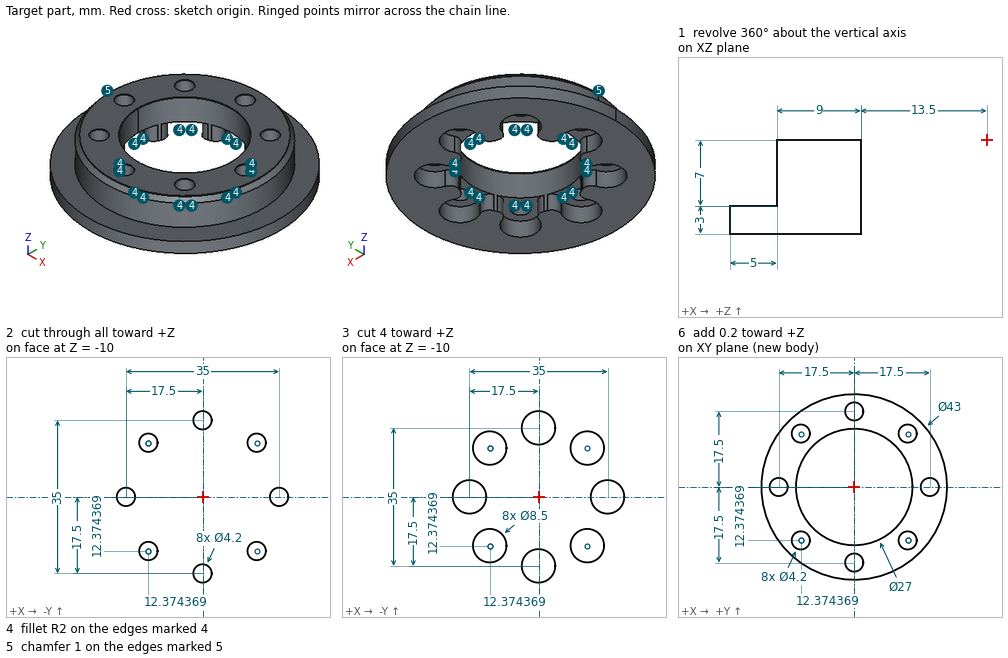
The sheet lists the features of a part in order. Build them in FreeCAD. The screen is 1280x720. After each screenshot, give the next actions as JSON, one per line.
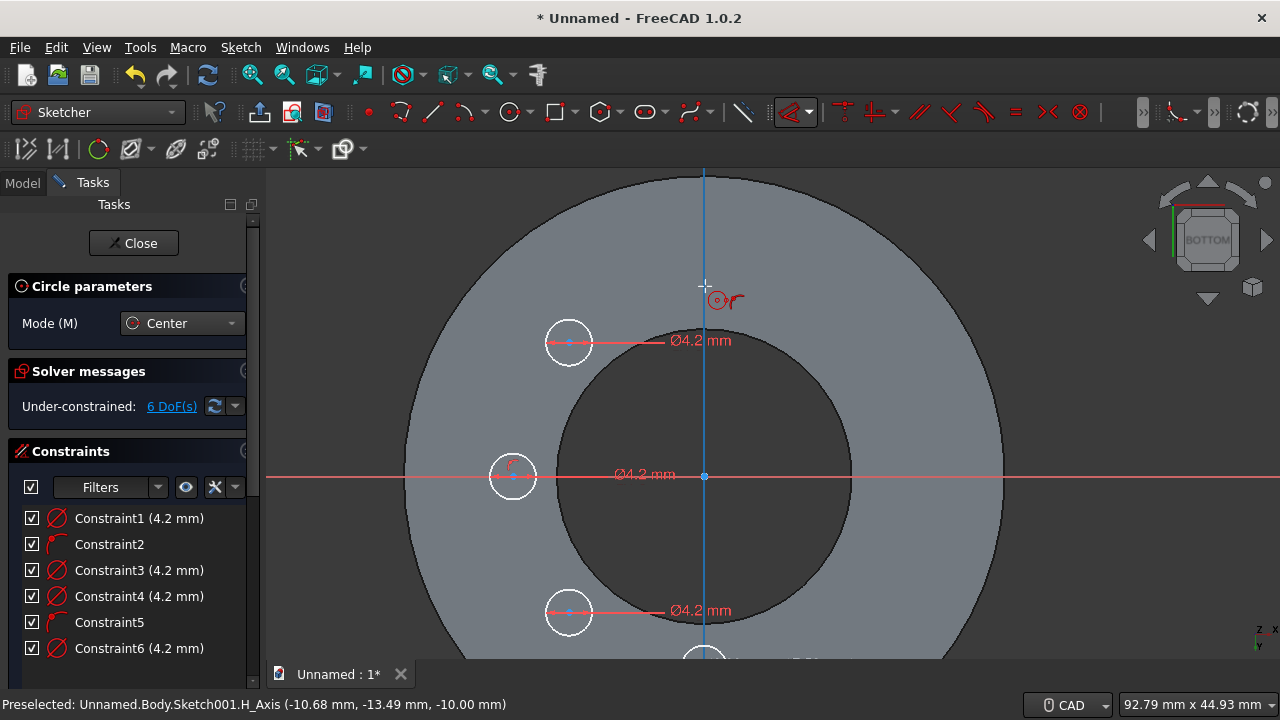
{"action": "left_click", "coordinate": [704, 285]}
{"action": "mouse_move", "coordinate": [720, 269]}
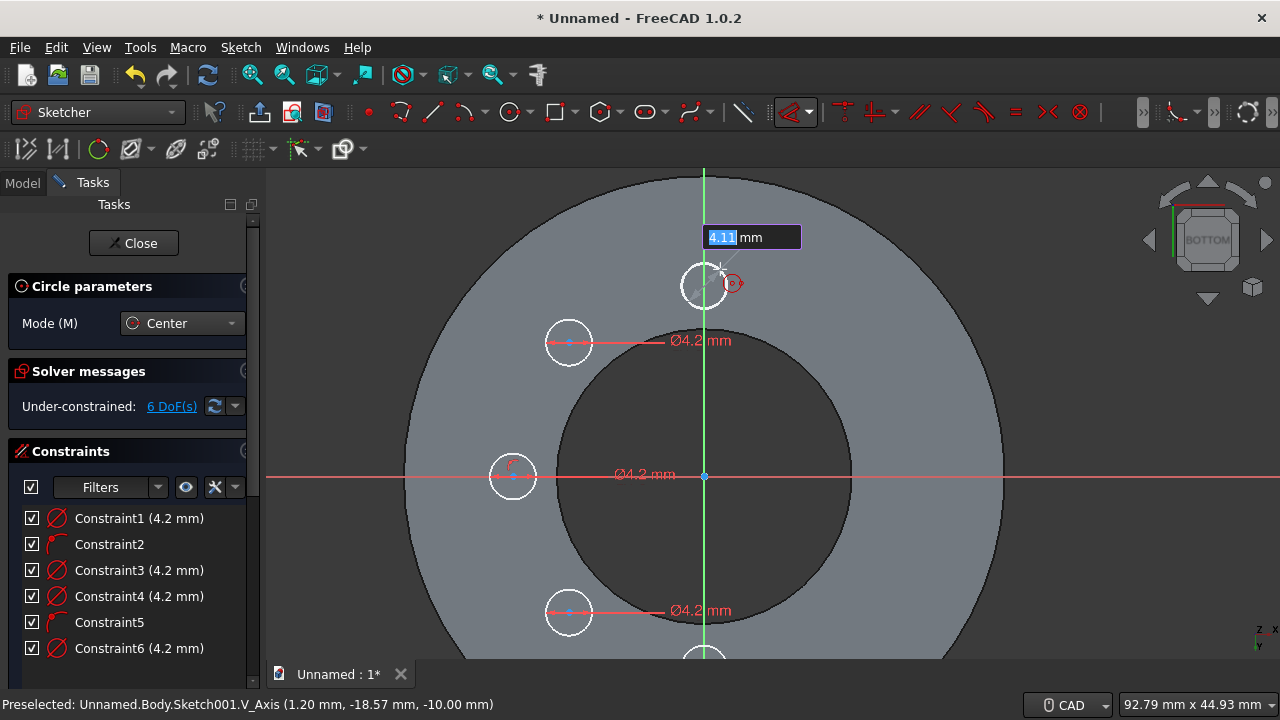
{"action": "type", "text": "4.2"}
{"action": "key", "text": "Return"}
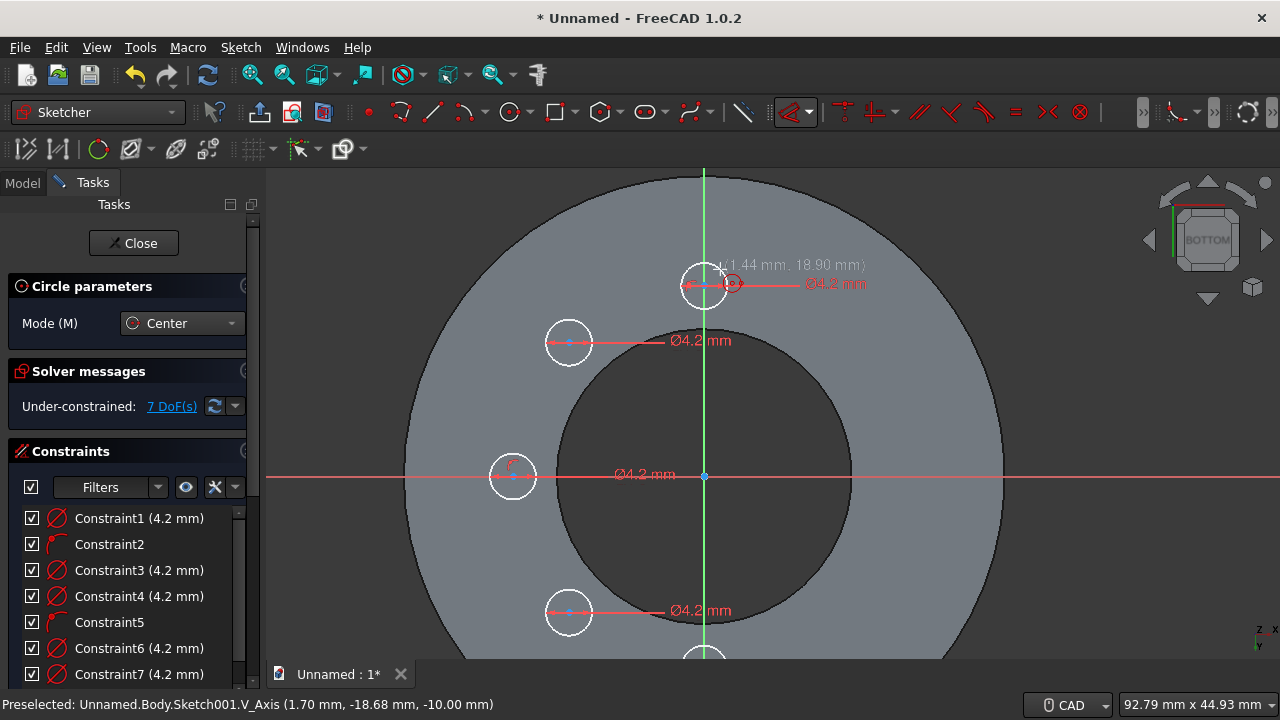
{"action": "left_click", "coordinate": [839, 341]}
{"action": "mouse_move", "coordinate": [856, 325]}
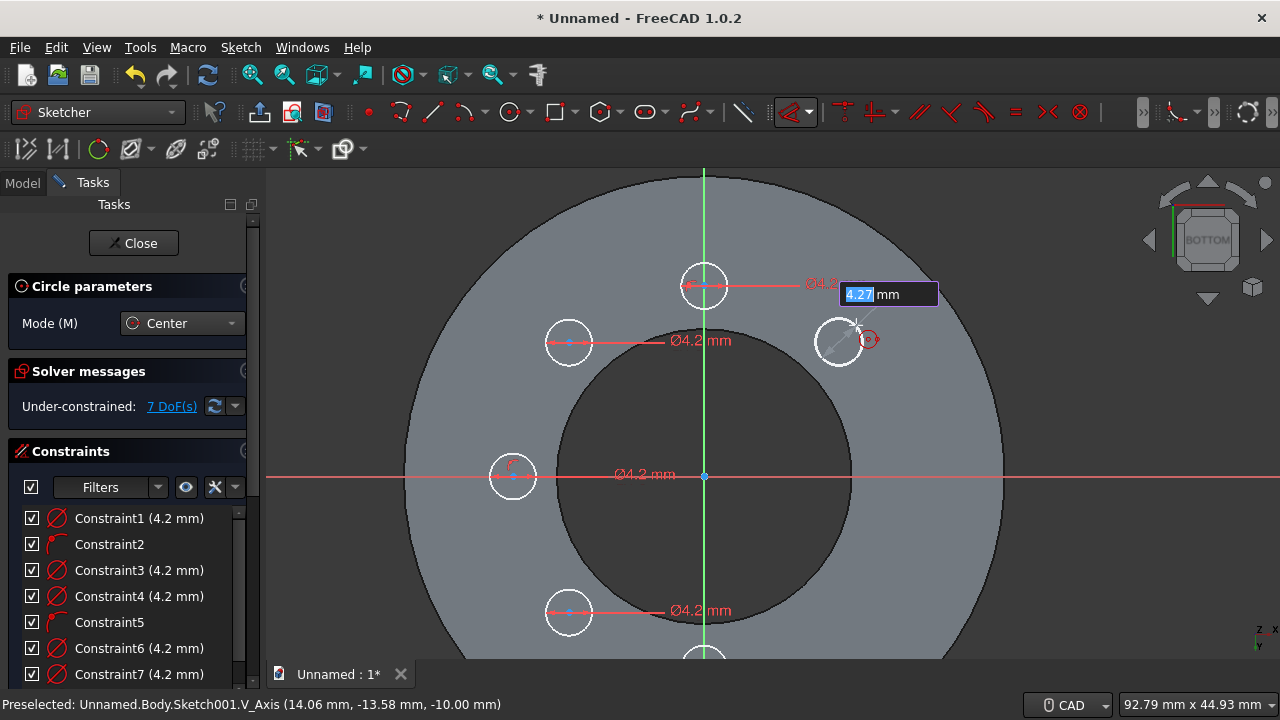
{"action": "type", "text": "4.2"}
{"action": "key", "text": "Return"}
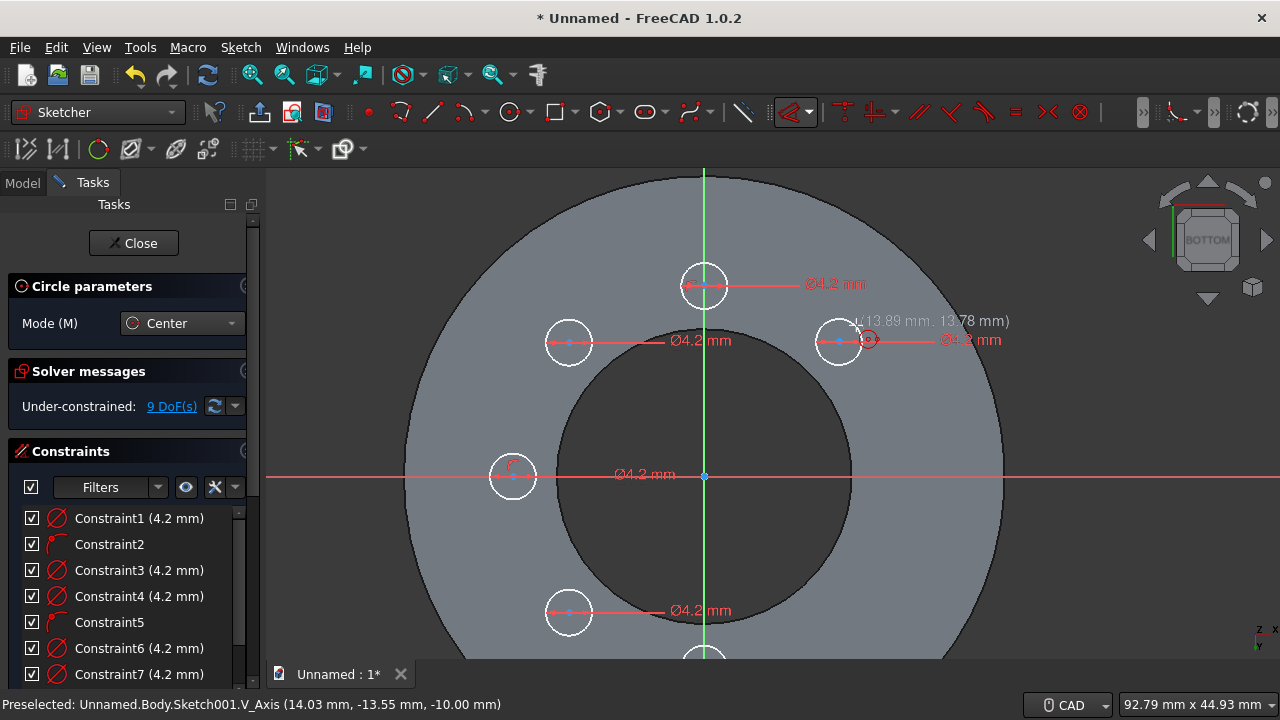
{"action": "left_click", "coordinate": [895, 477]}
{"action": "mouse_move", "coordinate": [912, 460]}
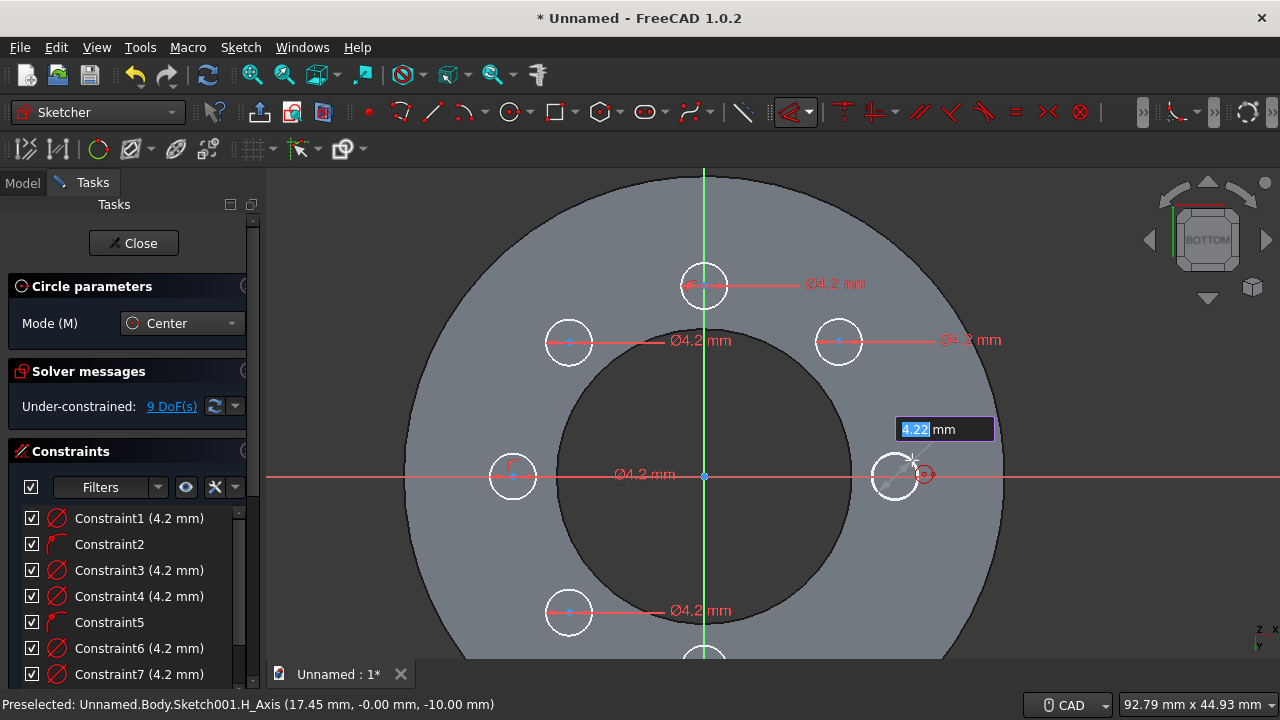
{"action": "type", "text": "4.2"}
{"action": "key", "text": "Return"}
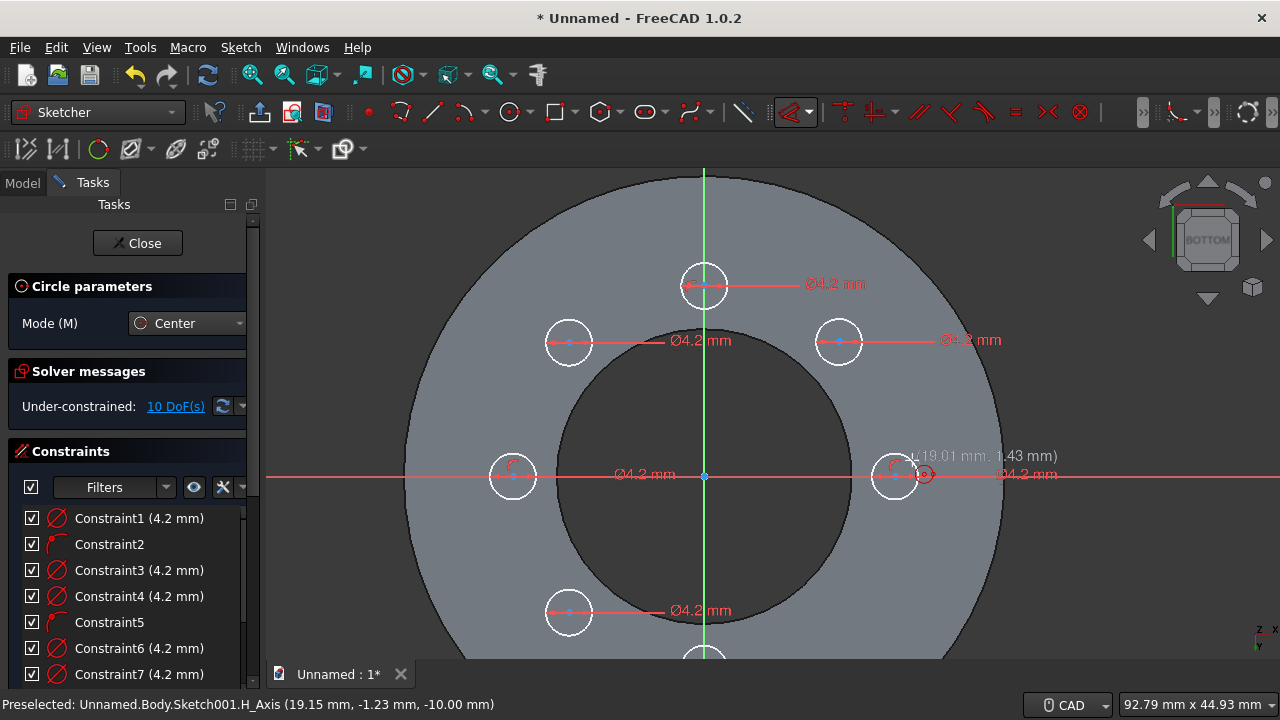
{"action": "left_click", "coordinate": [839, 612]}
{"action": "mouse_move", "coordinate": [856, 596]}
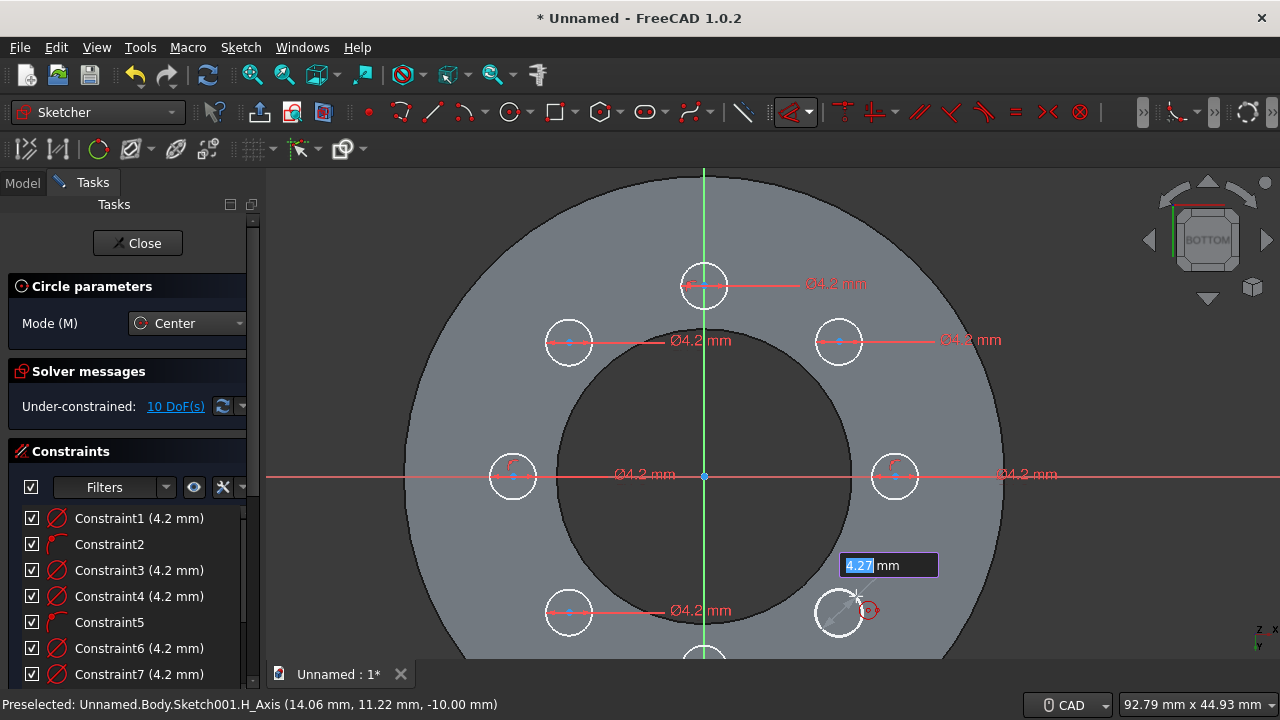
{"action": "type", "text": "4.2"}
{"action": "key", "text": "Return"}
{"action": "key", "text": "Escape"}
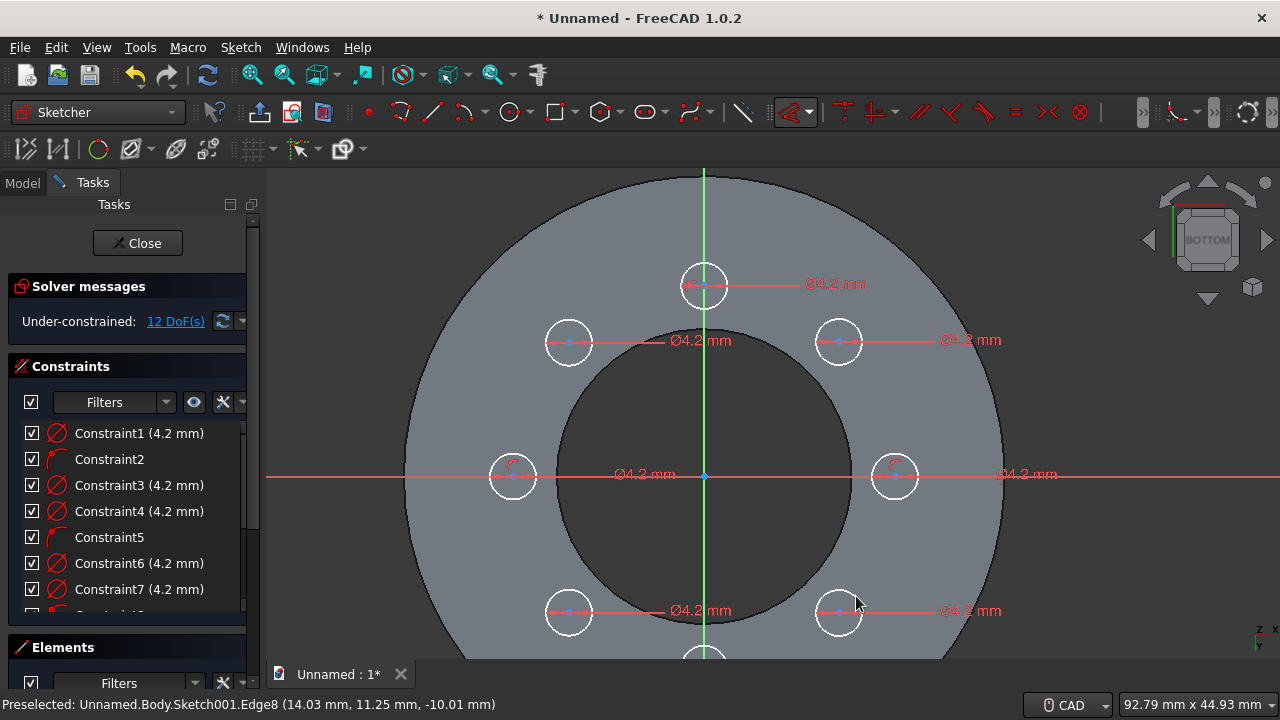
{"action": "left_click", "coordinate": [569, 613]}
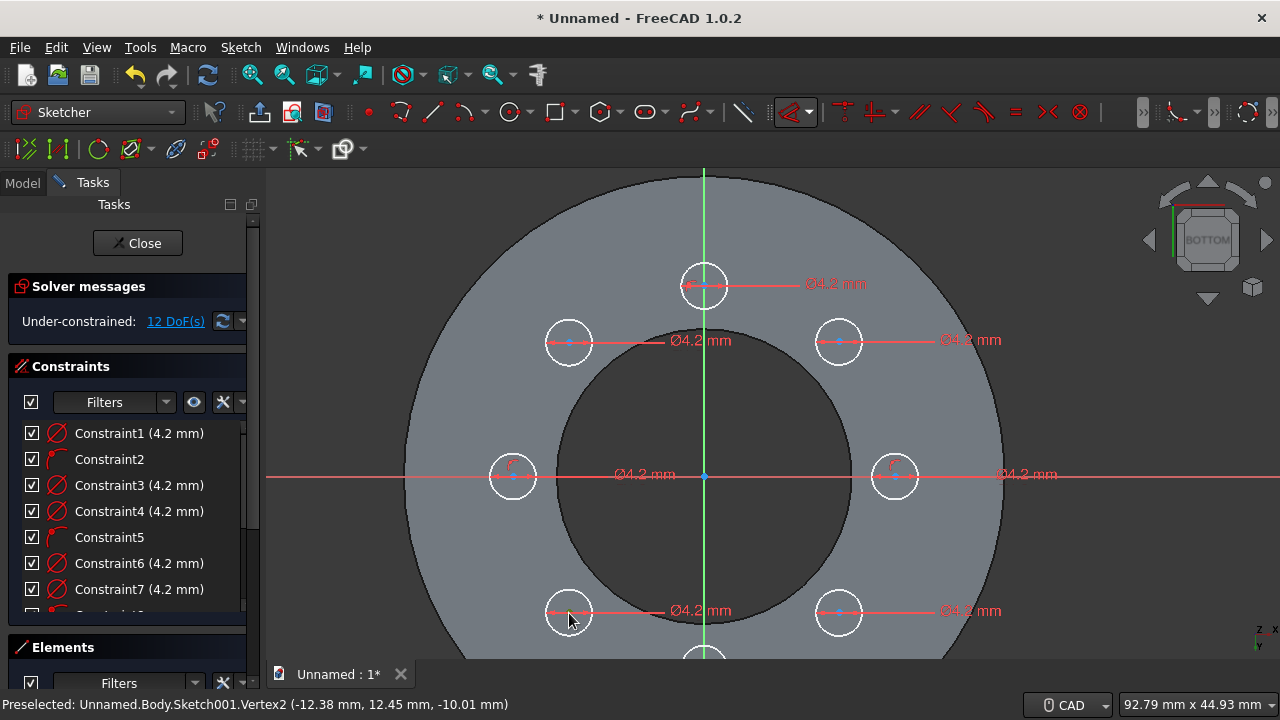
{"action": "left_click", "coordinate": [569, 343]}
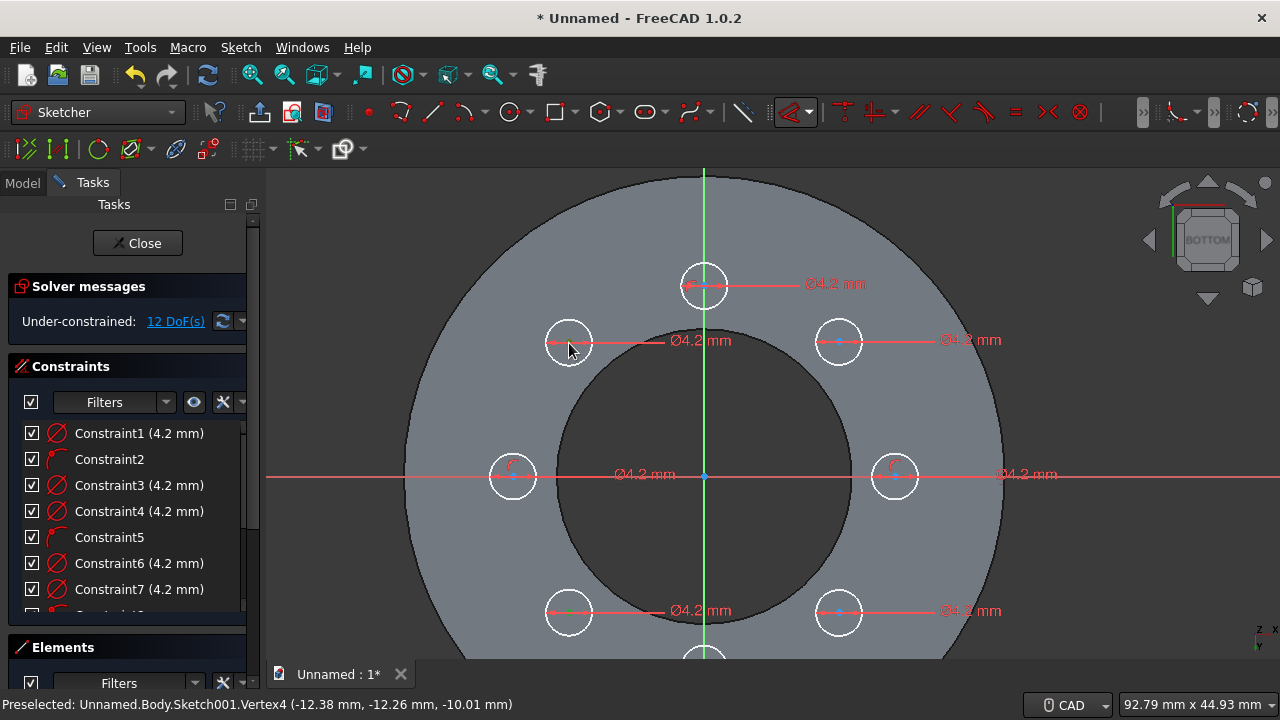
{"action": "left_click", "coordinate": [353, 477]}